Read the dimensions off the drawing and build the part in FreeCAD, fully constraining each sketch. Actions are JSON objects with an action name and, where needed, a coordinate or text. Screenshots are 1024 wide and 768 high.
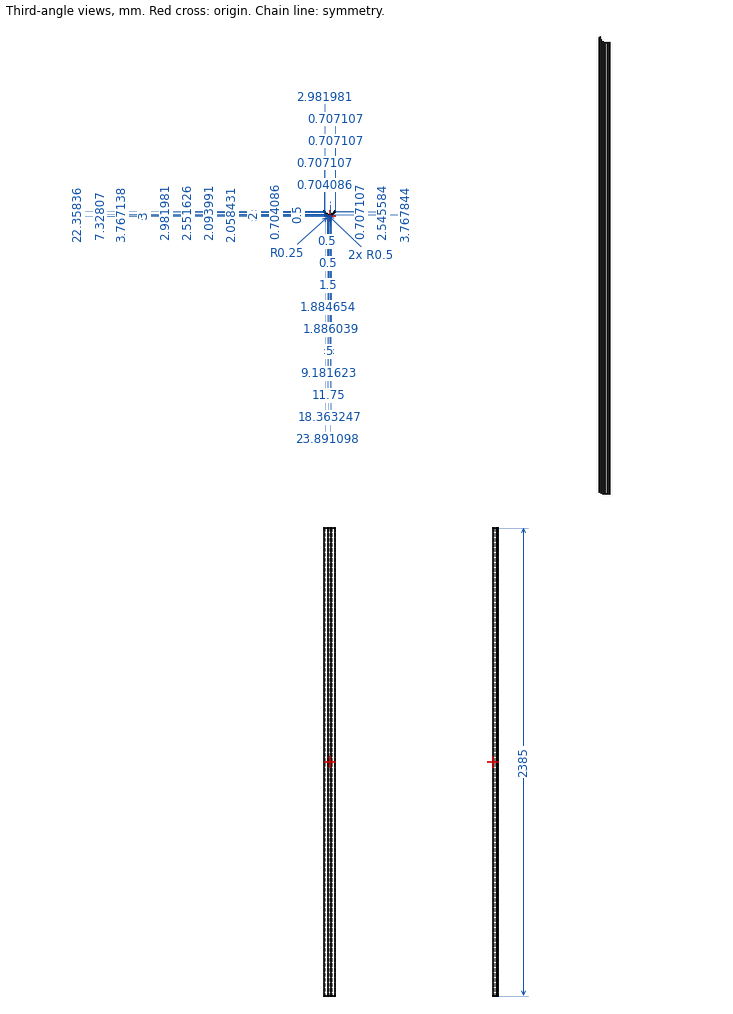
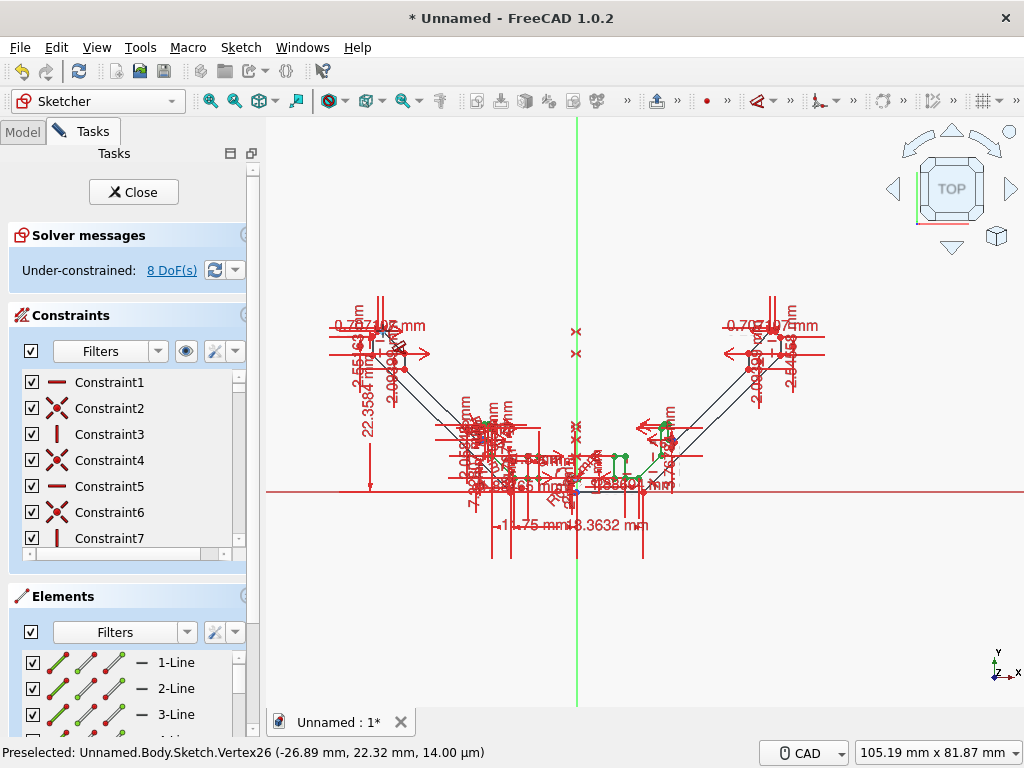
{"action": "left_click", "coordinate": [511, 492]}
{"action": "left_click", "coordinate": [544, 550]}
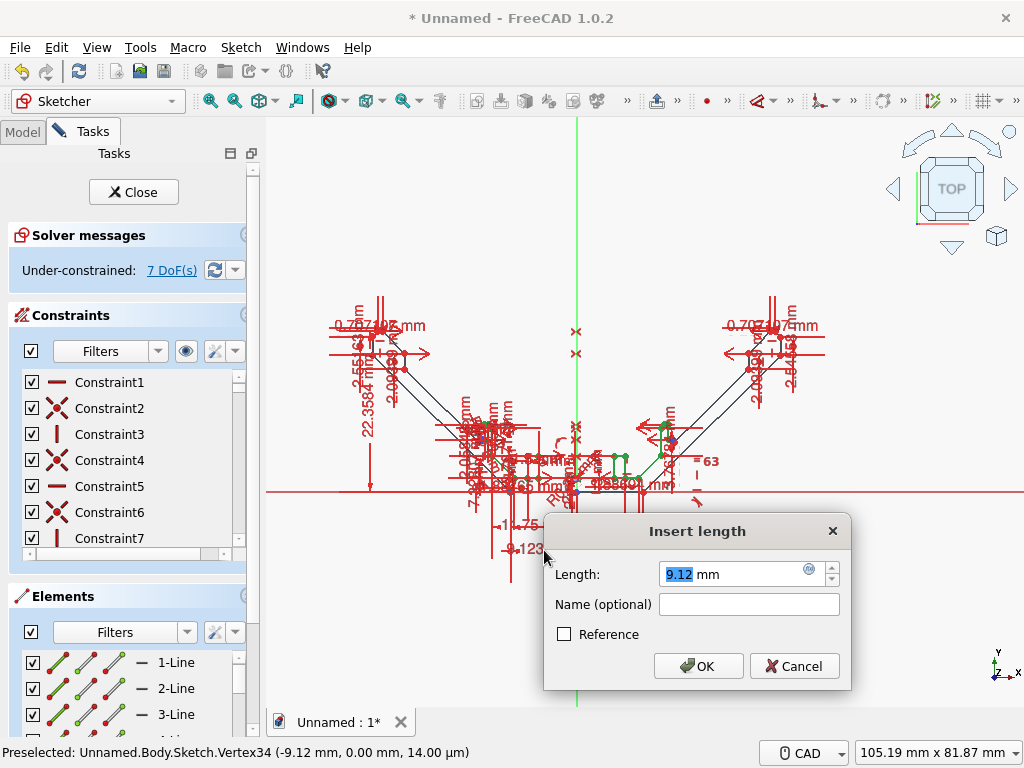
{"action": "type", "text": "9.181623"}
{"action": "key", "text": "Return"}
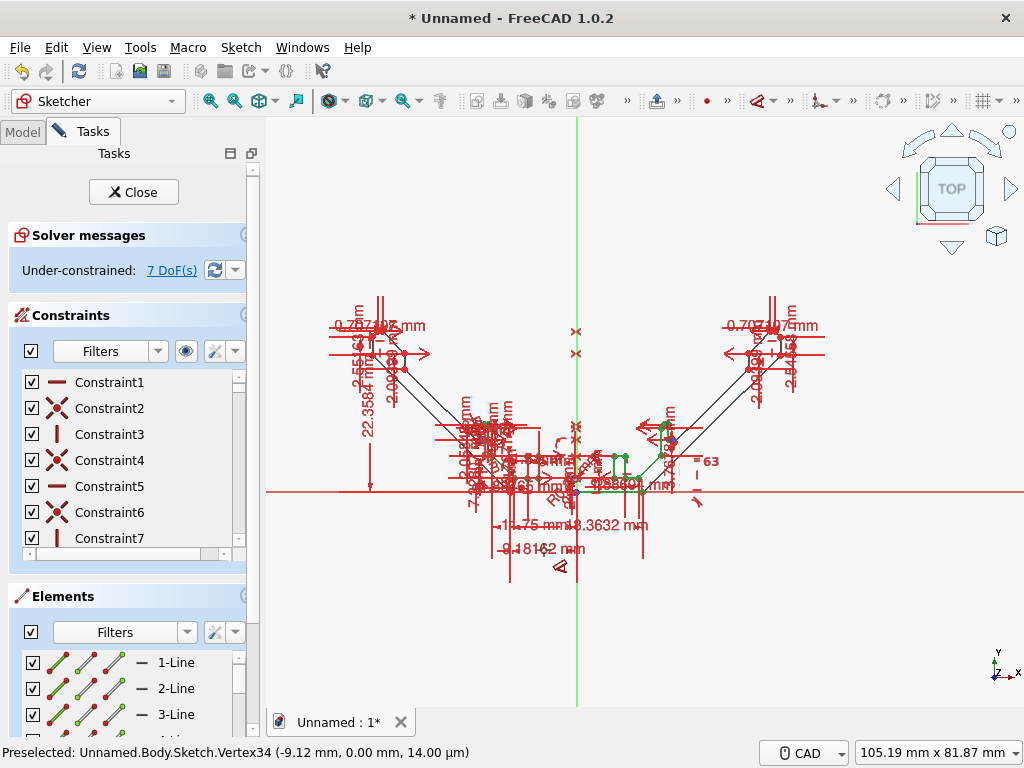
{"action": "scroll", "coordinate": [398, 347], "scroll_direction": "up", "scroll_amount": 4}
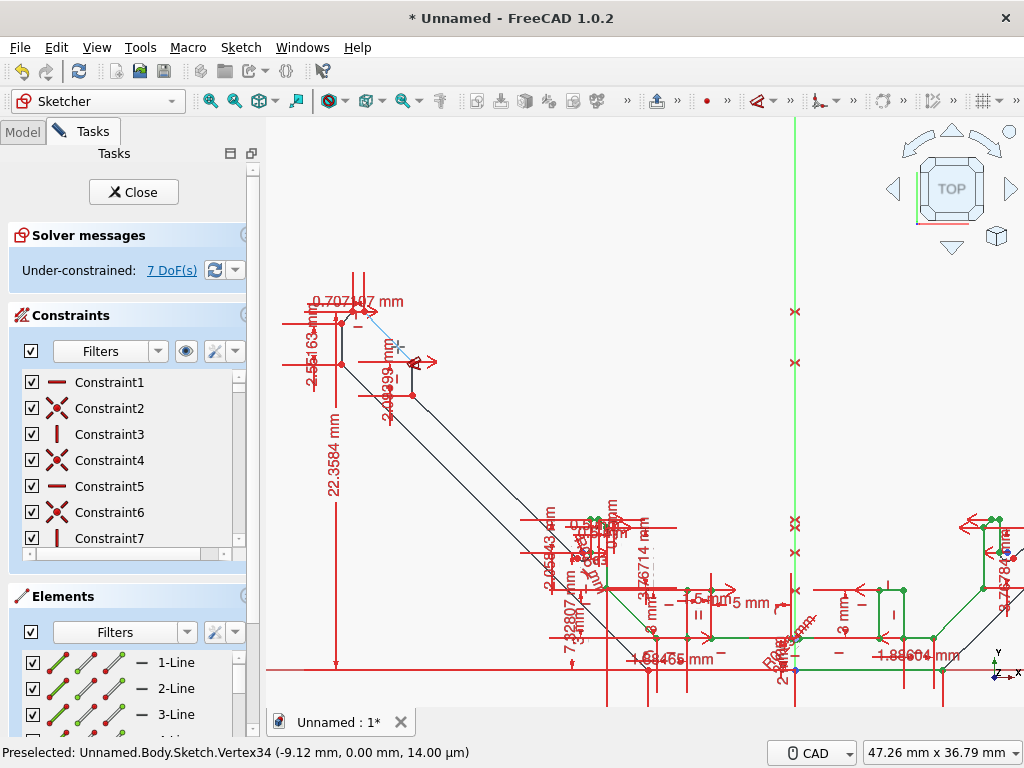
{"action": "left_click", "coordinate": [398, 347]}
{"action": "left_click", "coordinate": [388, 278]}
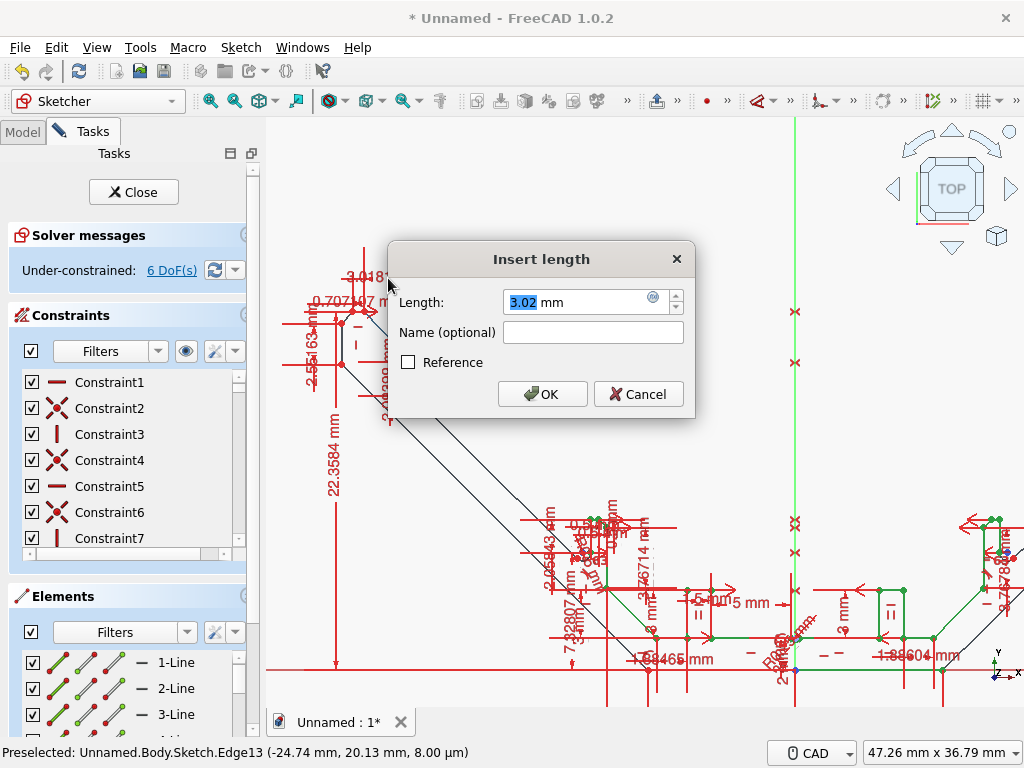
{"action": "type", "text": "2.981981"}
{"action": "key", "text": "Return"}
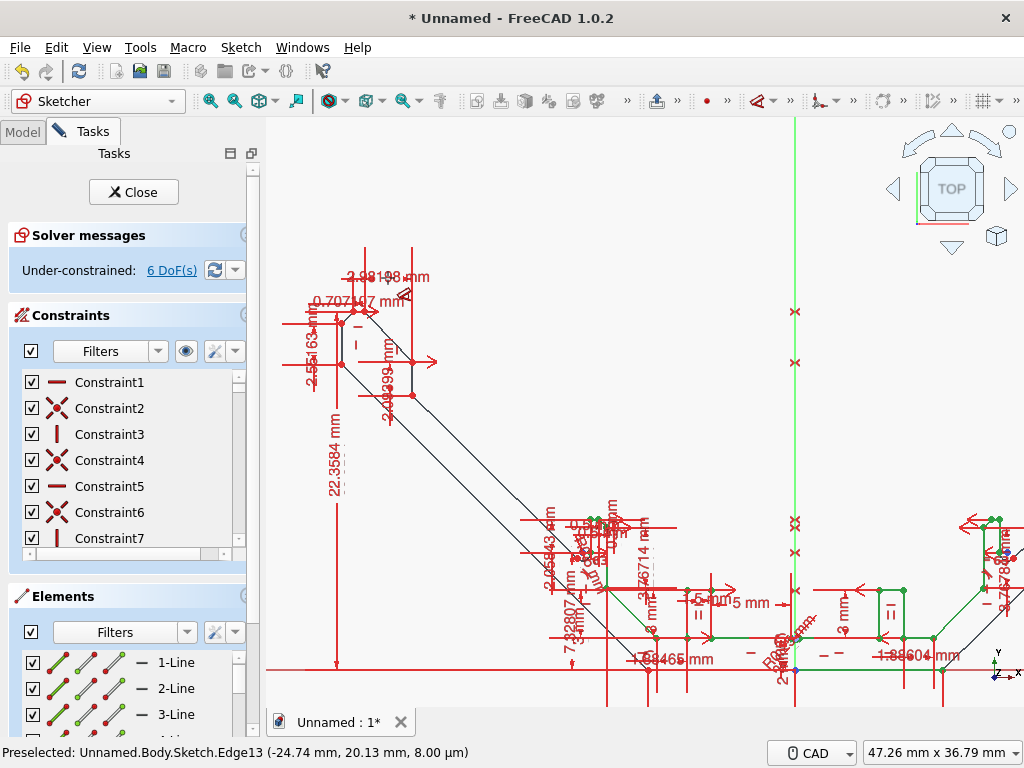
{"action": "left_click", "coordinate": [398, 347]}
{"action": "left_click", "coordinate": [446, 337]}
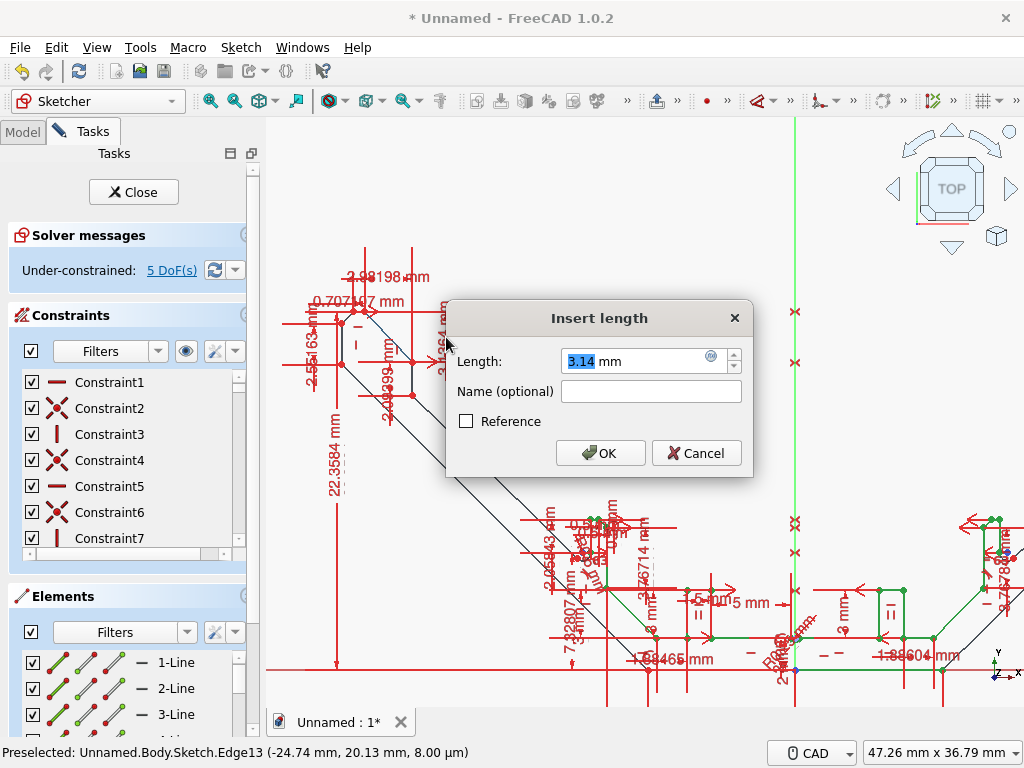
{"action": "type", "text": "2.981981"}
{"action": "key", "text": "Return"}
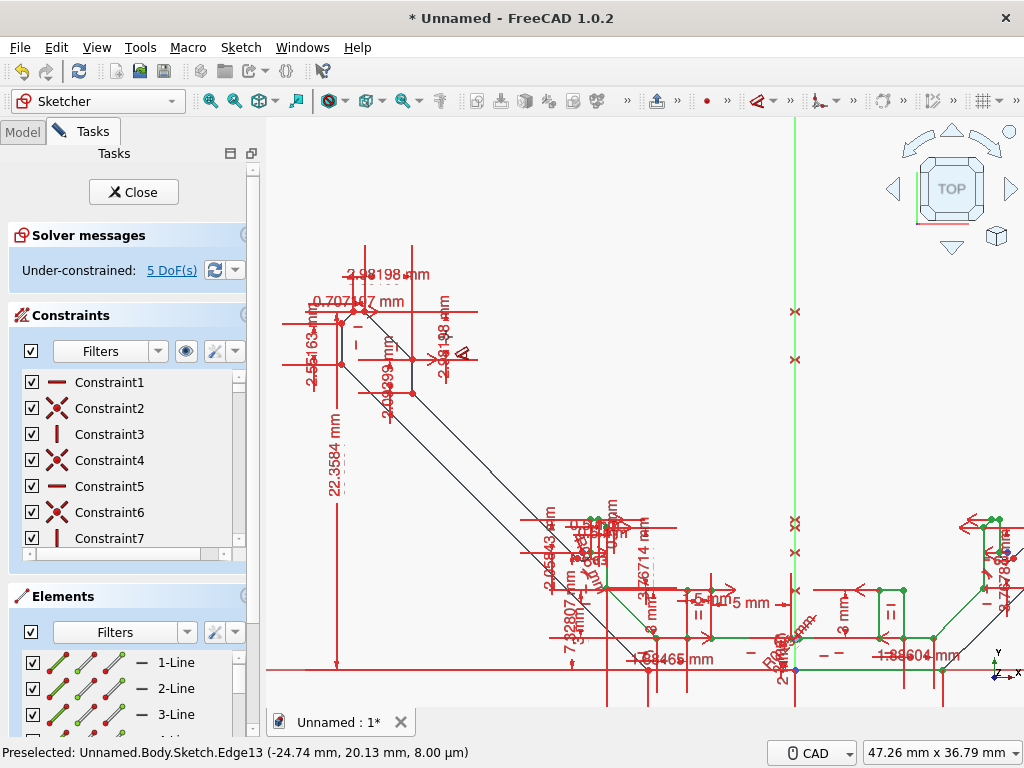
{"action": "scroll", "coordinate": [348, 318], "scroll_direction": "up", "scroll_amount": 7}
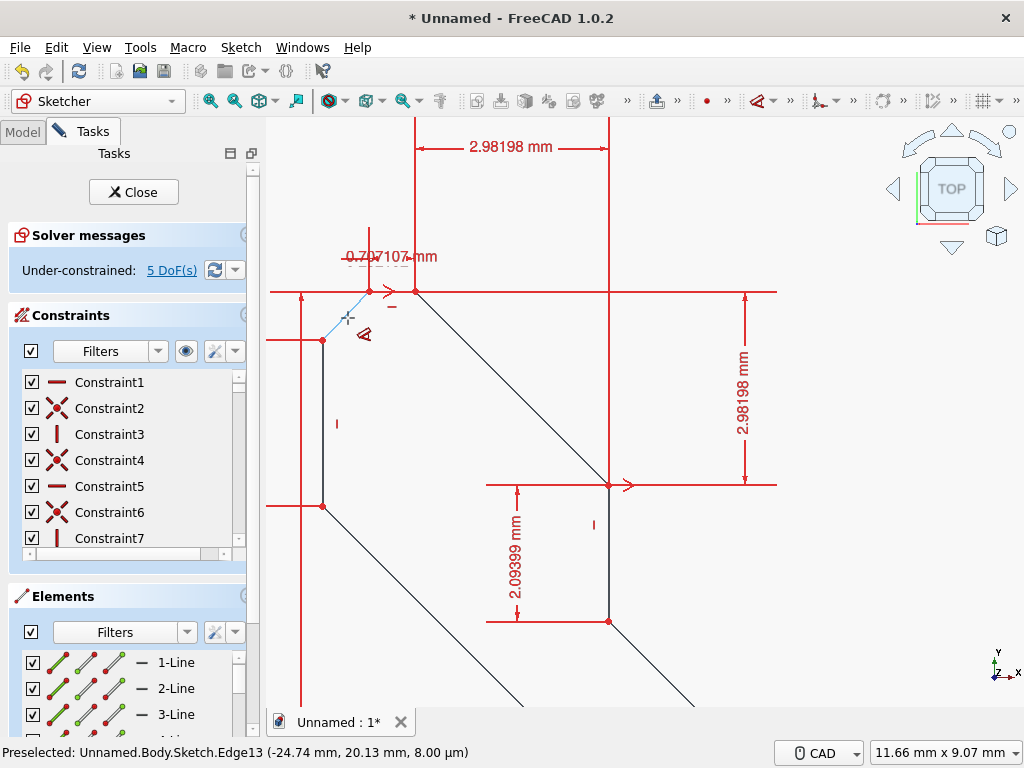
{"action": "left_click", "coordinate": [346, 316]}
{"action": "left_click", "coordinate": [346, 374]}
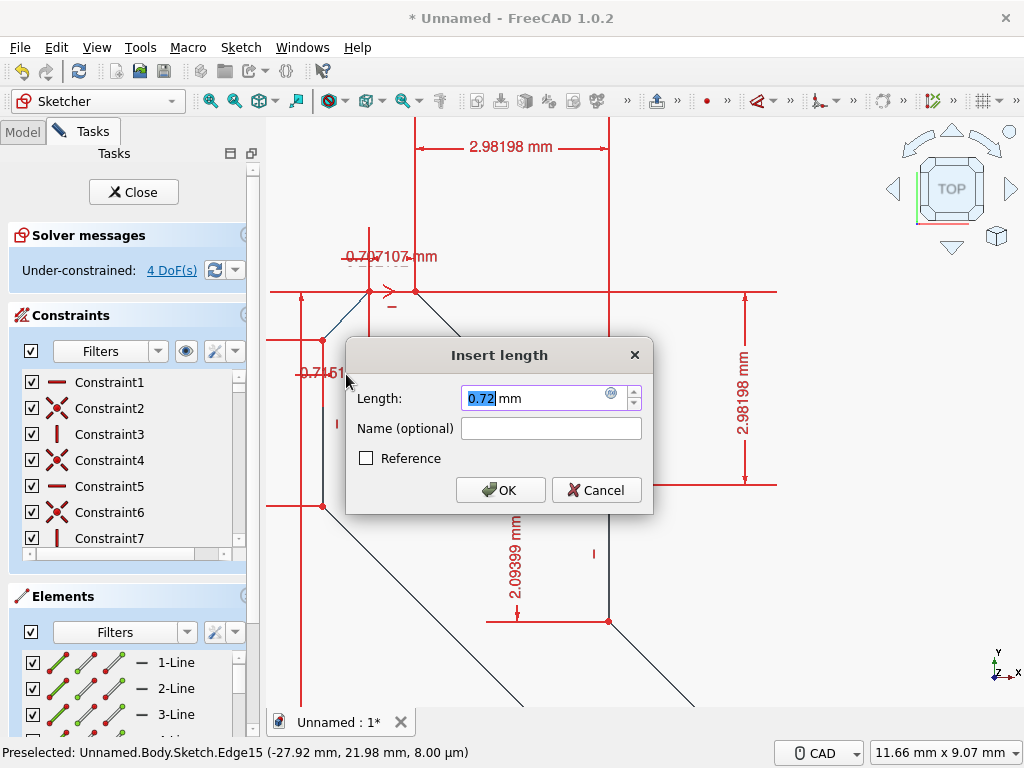
{"action": "type", "text": "0.704086"}
{"action": "key", "text": "Return"}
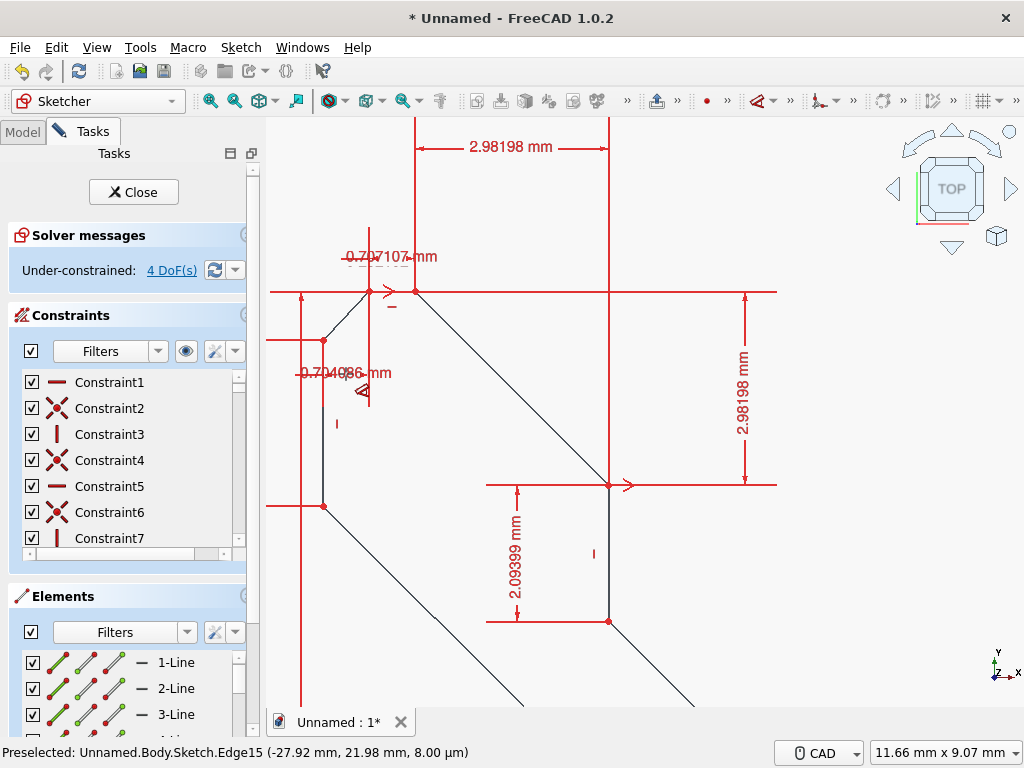
{"action": "left_click", "coordinate": [355, 306]}
{"action": "left_click", "coordinate": [403, 316]}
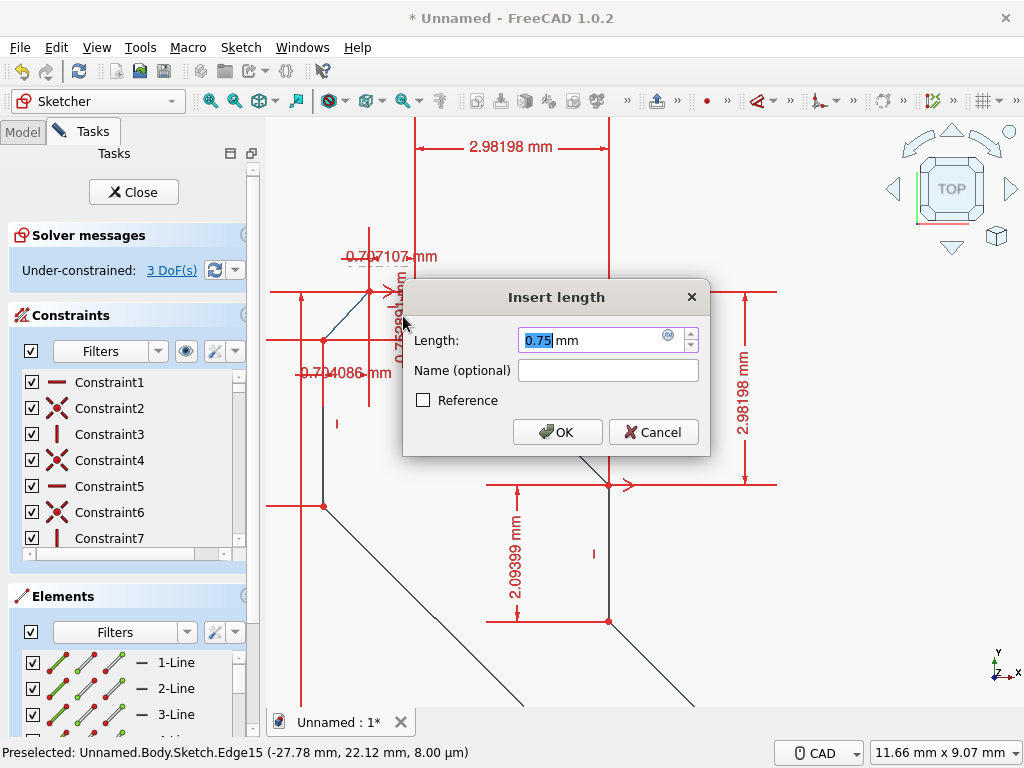
{"action": "type", "text": "0.704086"}
{"action": "key", "text": "Return"}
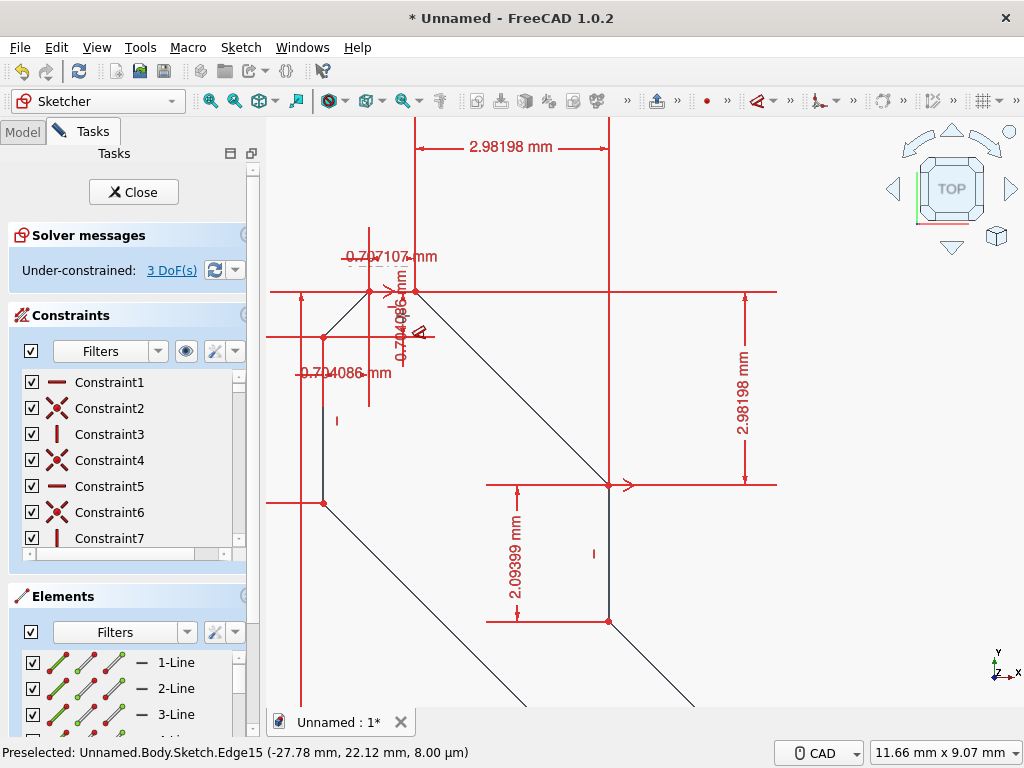
{"action": "scroll", "coordinate": [379, 336], "scroll_direction": "down", "scroll_amount": 11}